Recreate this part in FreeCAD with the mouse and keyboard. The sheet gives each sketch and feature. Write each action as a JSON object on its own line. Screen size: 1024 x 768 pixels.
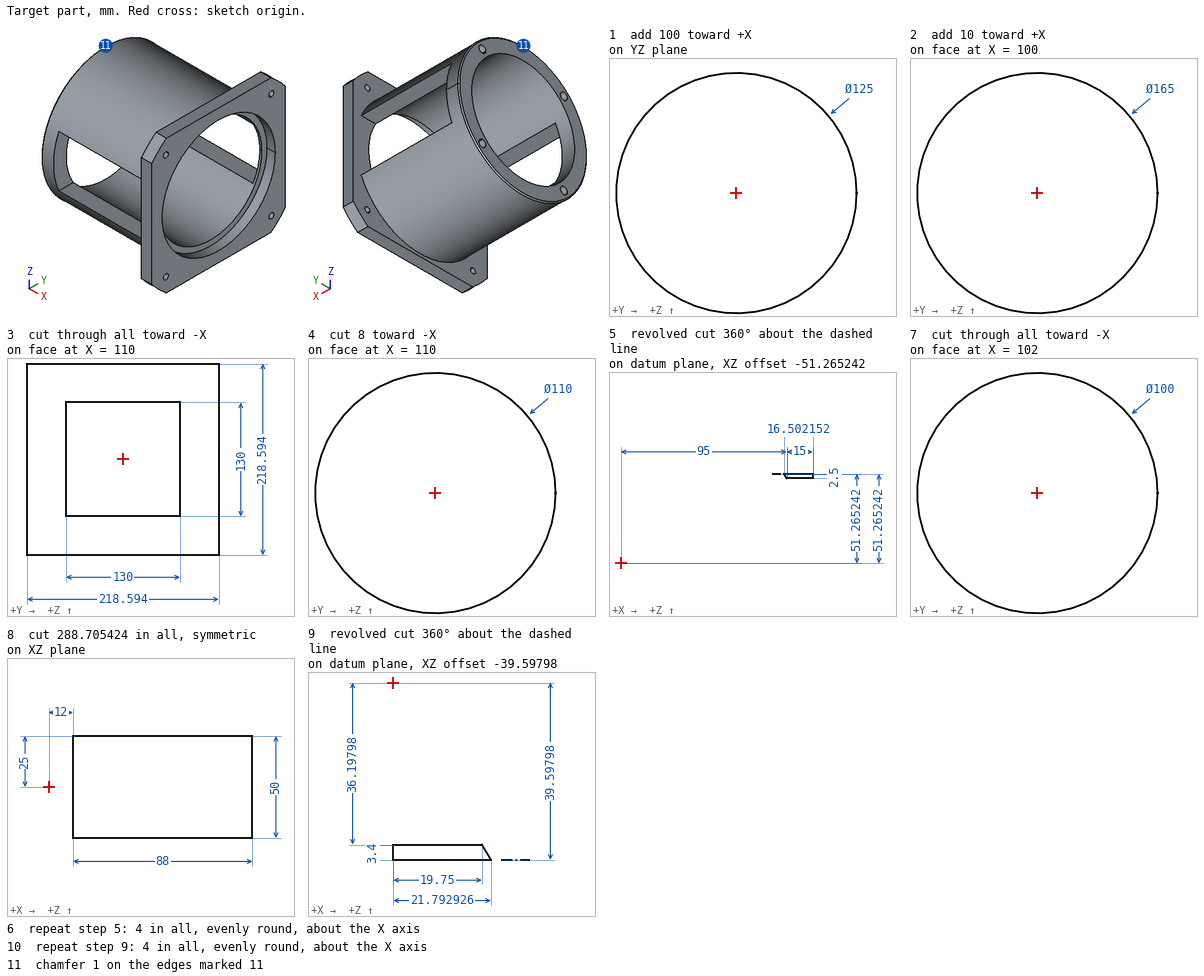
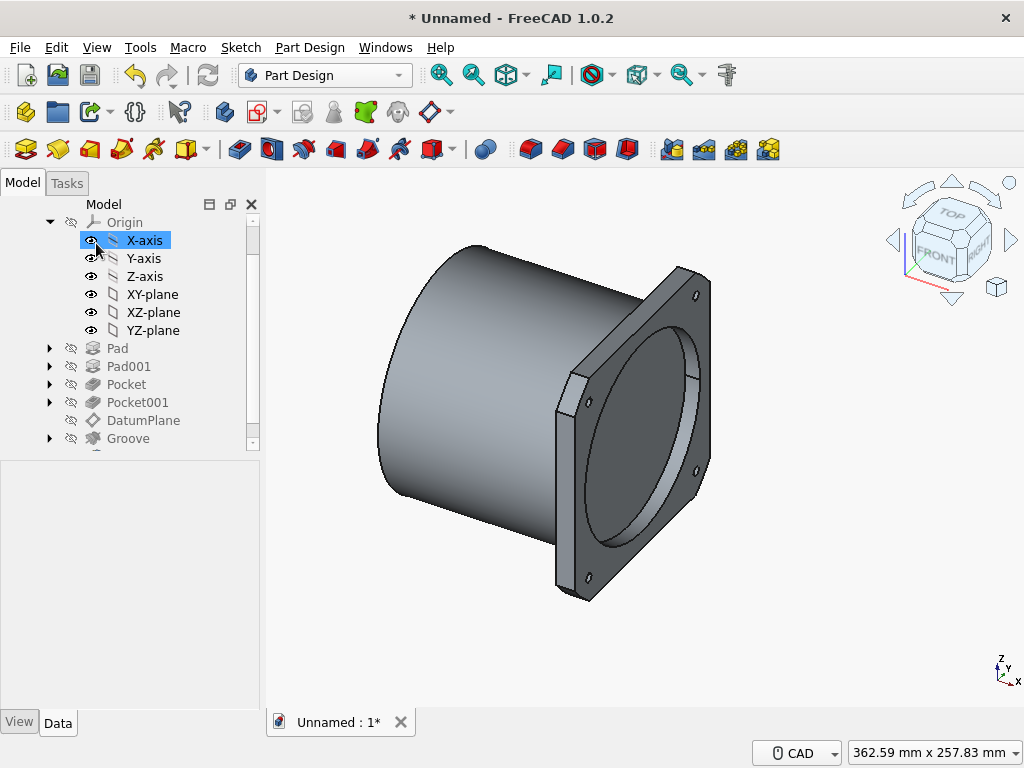
{"action": "left_click", "coordinate": [628, 431]}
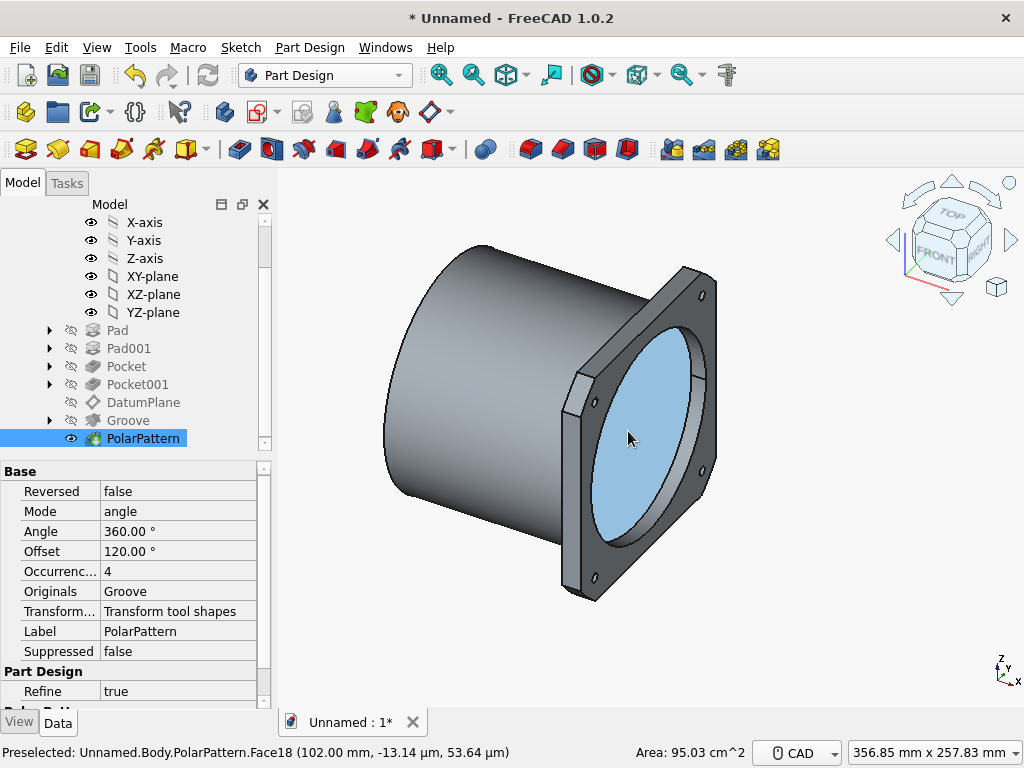
{"action": "left_click", "coordinate": [258, 112]}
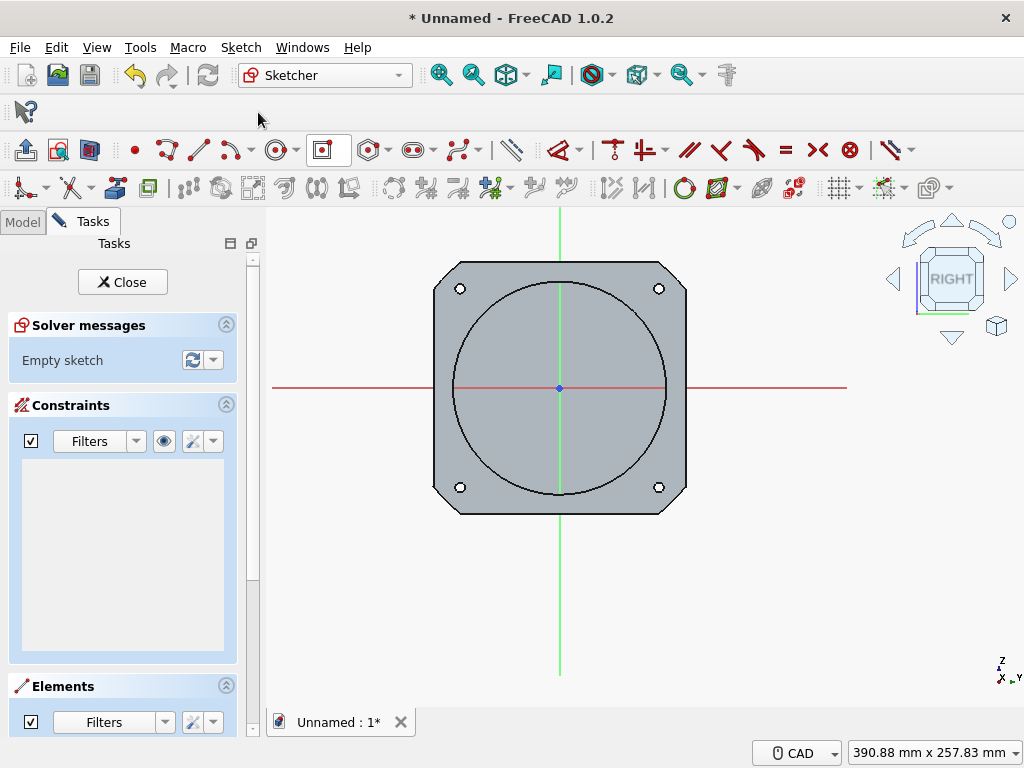
{"action": "scroll", "coordinate": [525, 248], "scroll_direction": "up", "scroll_amount": 2}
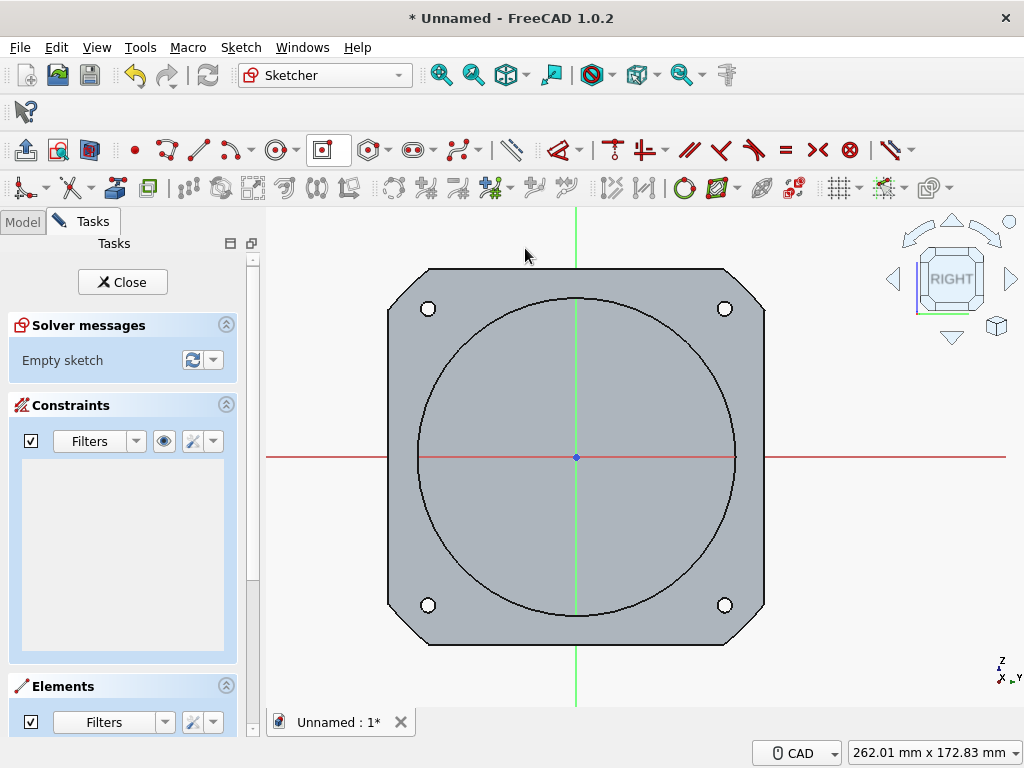
{"action": "left_click", "coordinate": [276, 150]}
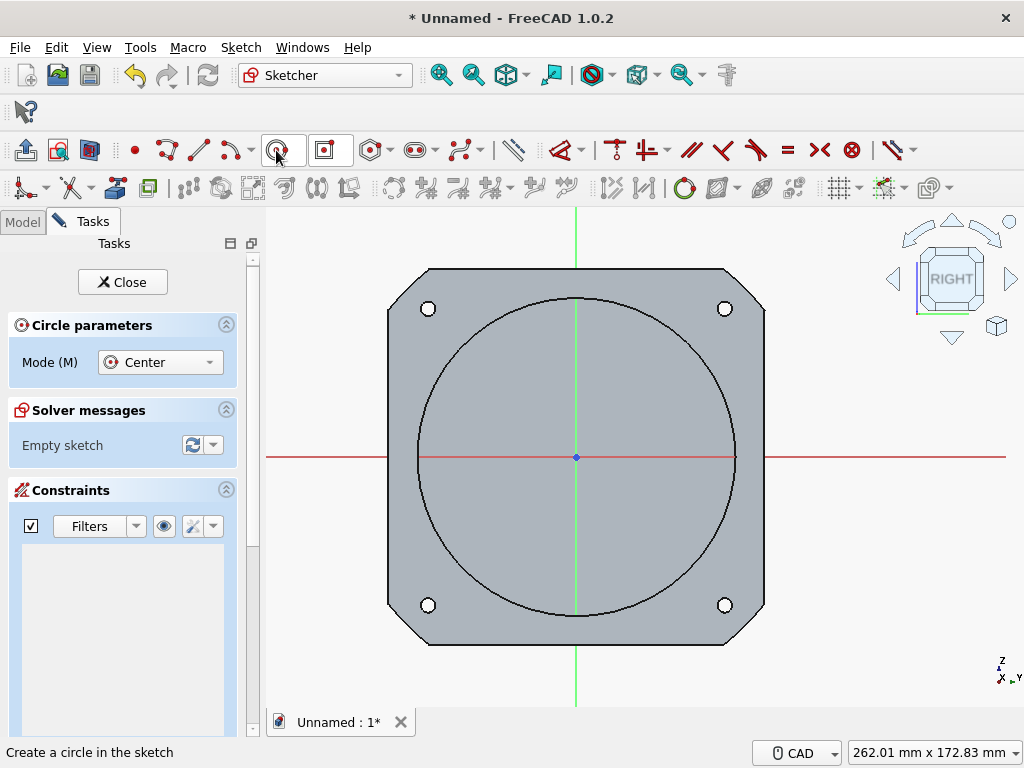
{"action": "left_click", "coordinate": [576, 457]}
{"action": "mouse_move", "coordinate": [679, 355]}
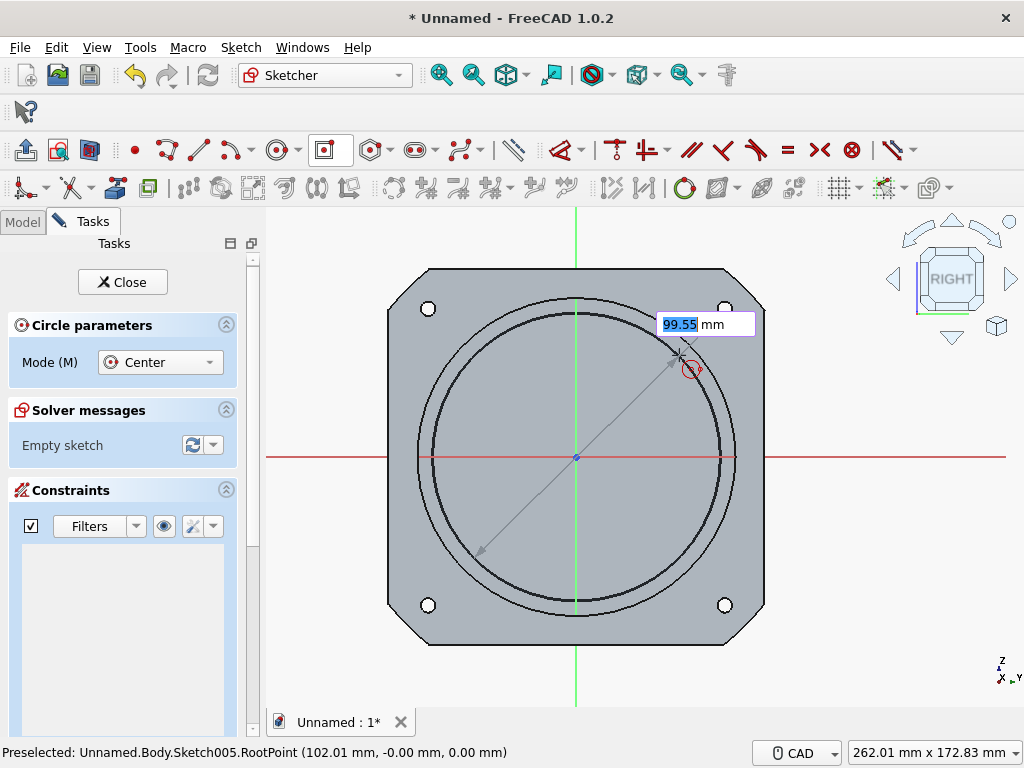
{"action": "type", "text": "100"}
{"action": "key", "text": "Return"}
{"action": "key", "text": "Escape"}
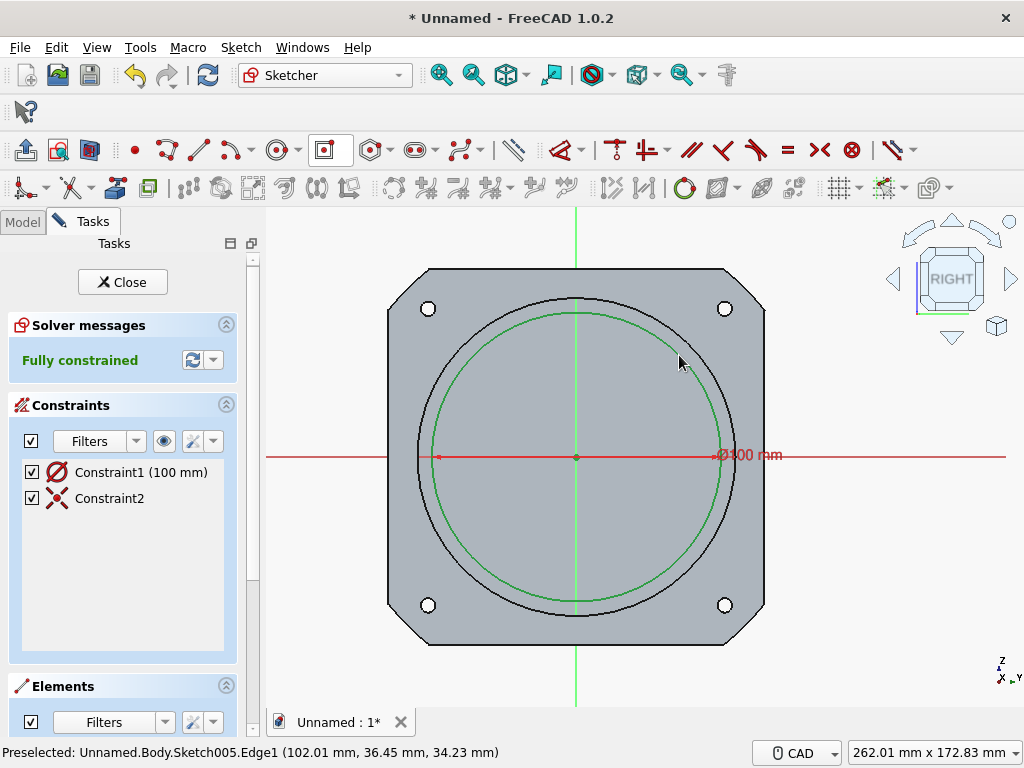
{"action": "left_click", "coordinate": [123, 282]}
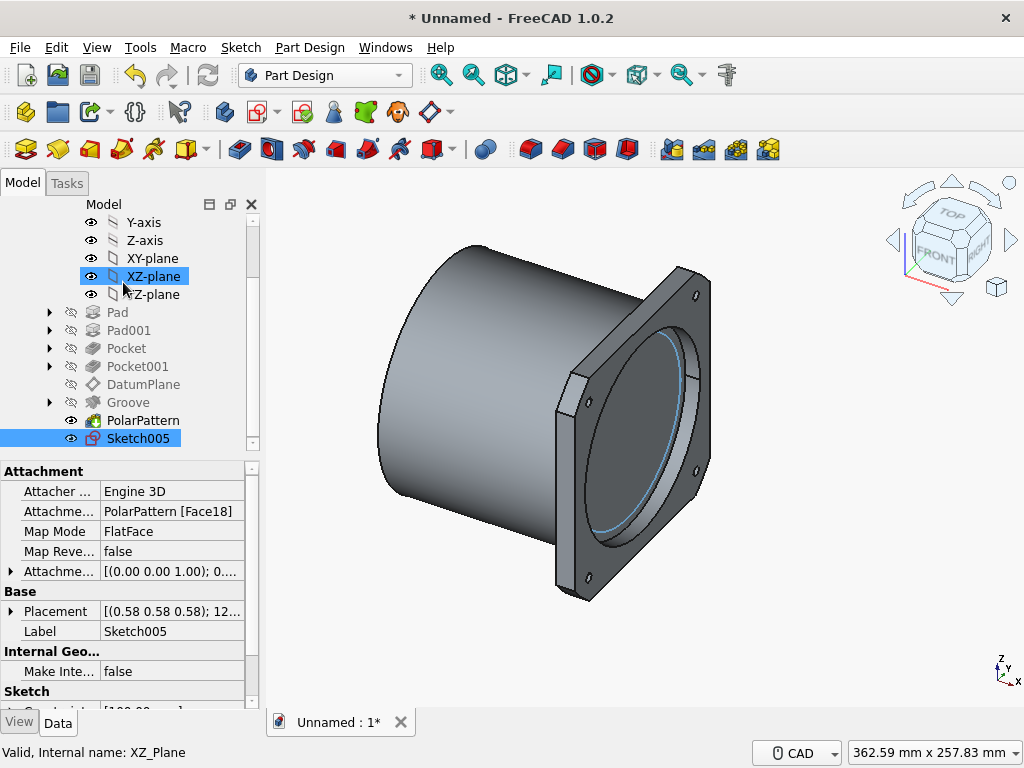
{"action": "left_click", "coordinate": [240, 150]}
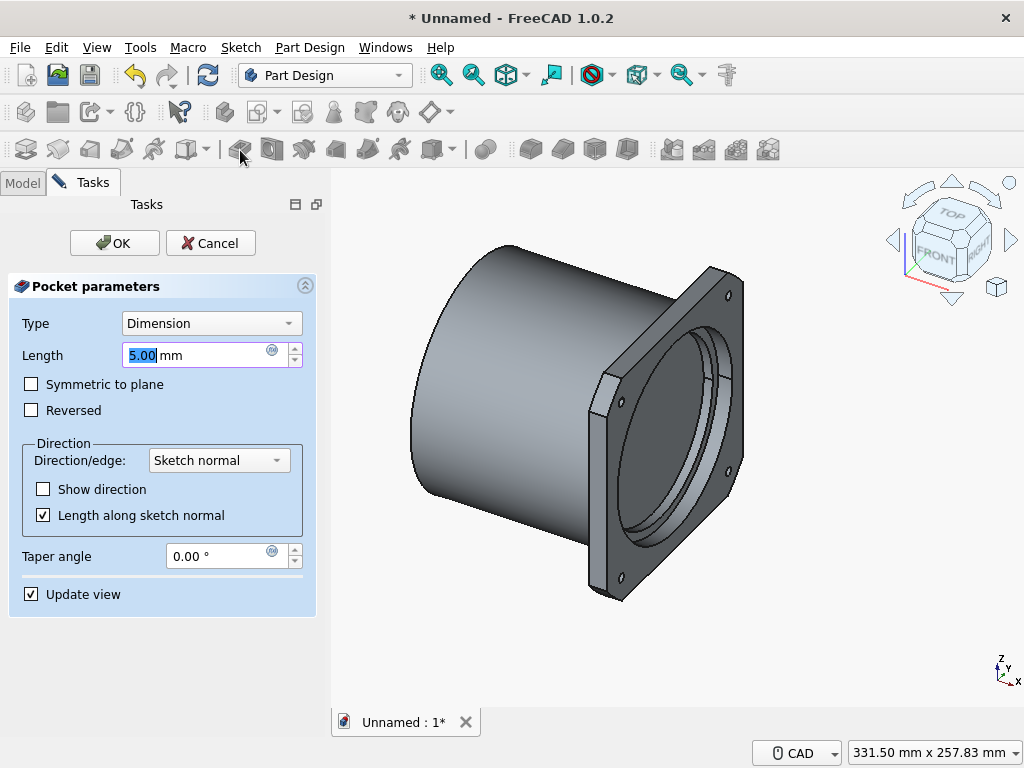
{"action": "left_click", "coordinate": [212, 324]}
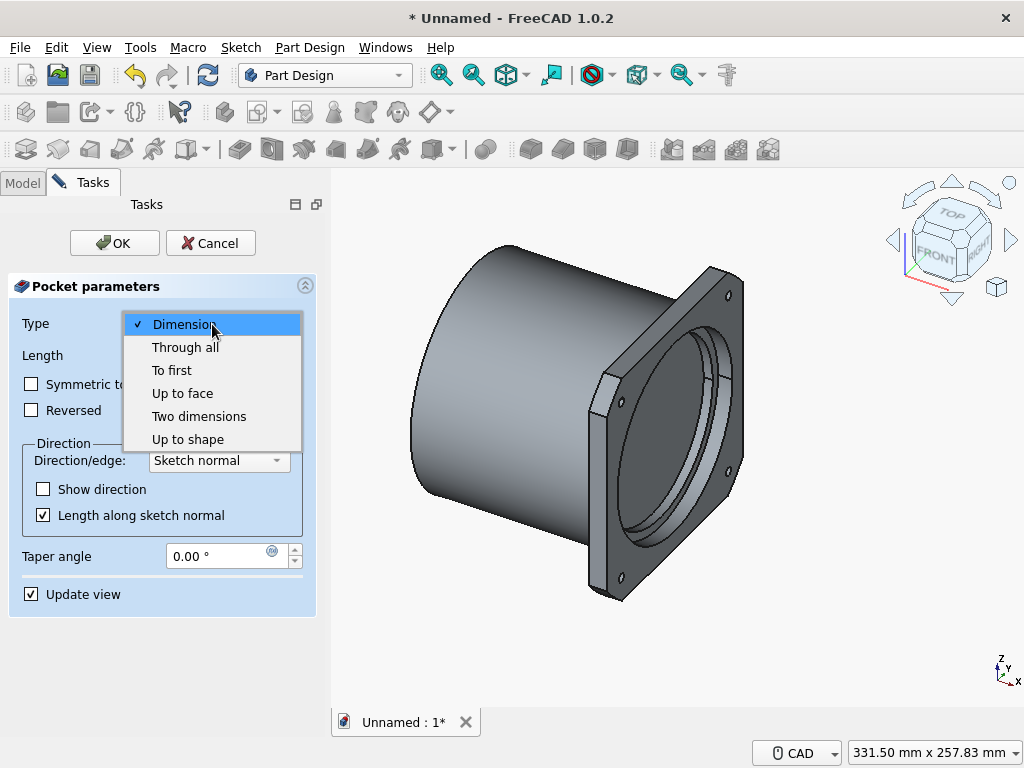
{"action": "left_click", "coordinate": [212, 348]}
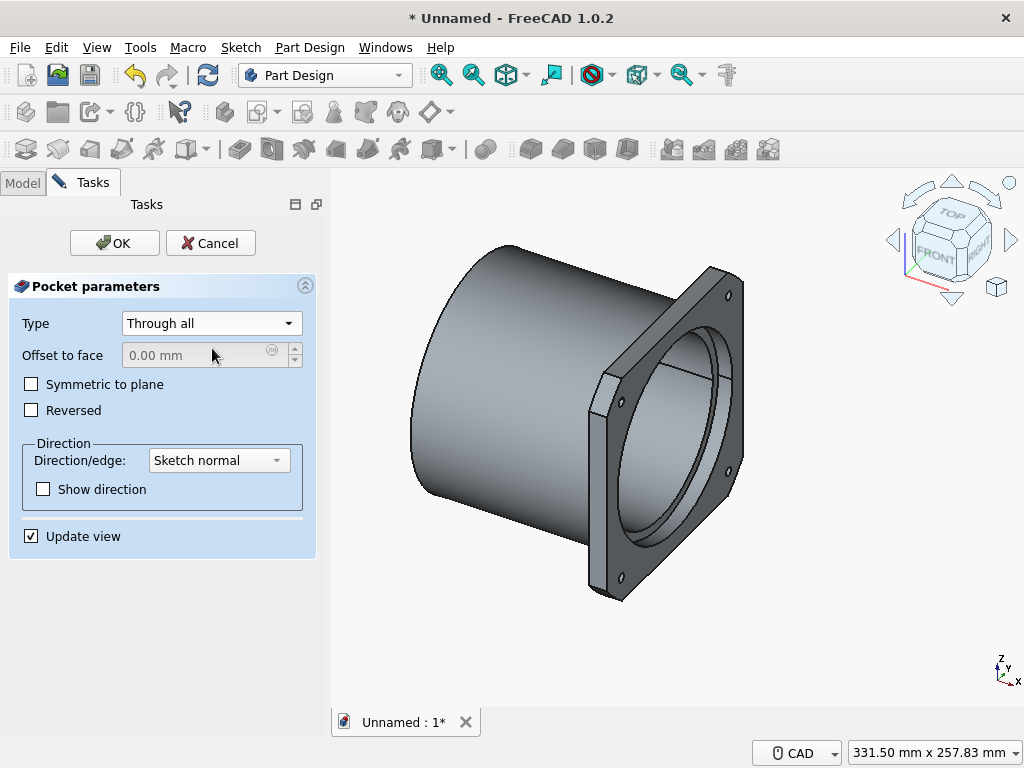
{"action": "left_click", "coordinate": [115, 243]}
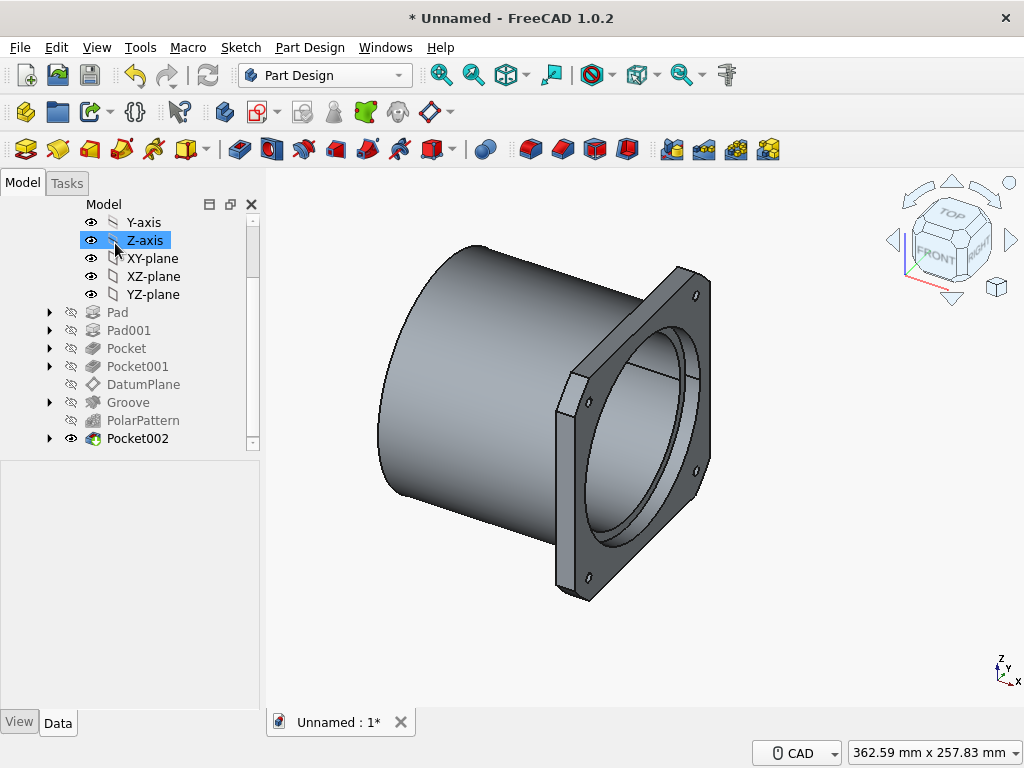
{"action": "left_click", "coordinate": [258, 112]}